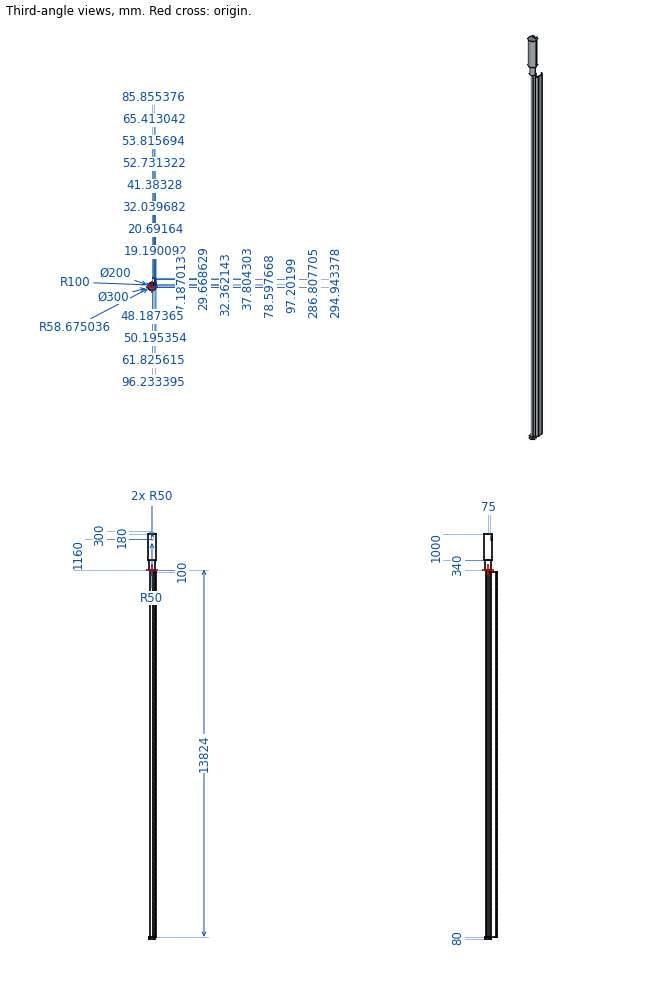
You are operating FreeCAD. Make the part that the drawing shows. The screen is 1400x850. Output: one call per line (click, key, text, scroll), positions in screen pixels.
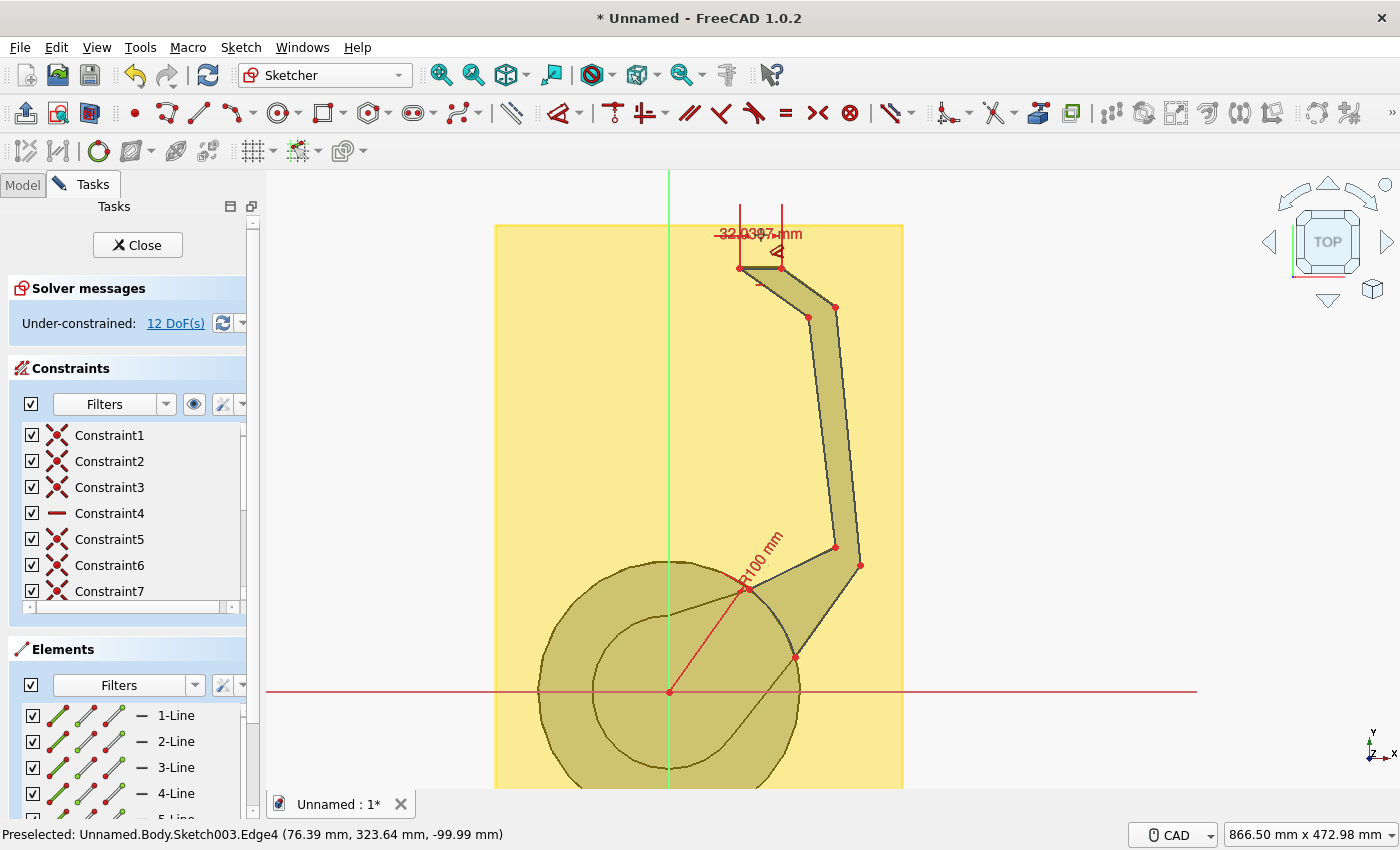
click(861, 566)
click(635, 629)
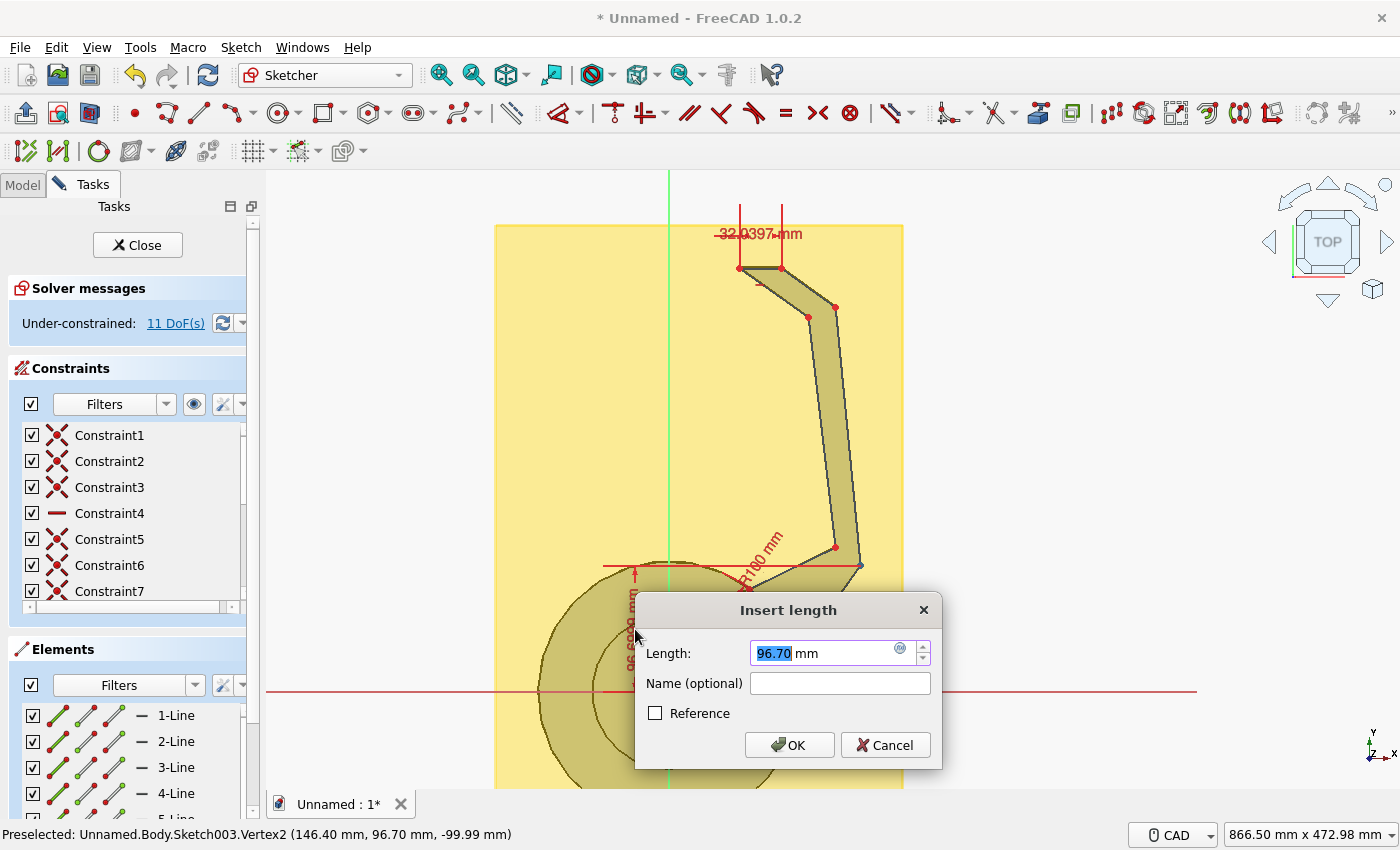
text(97.20199)
key(Return)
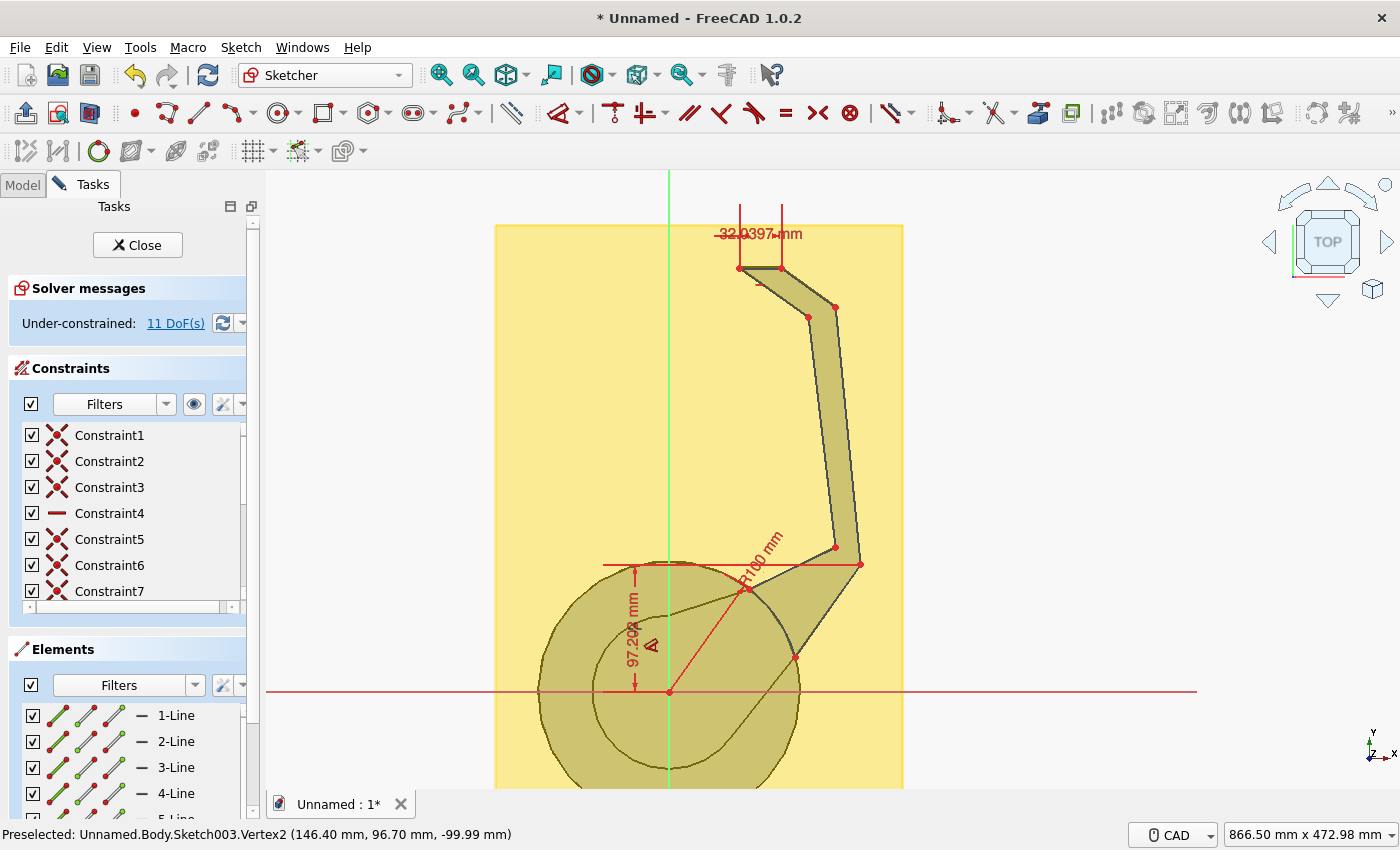
click(819, 296)
click(796, 342)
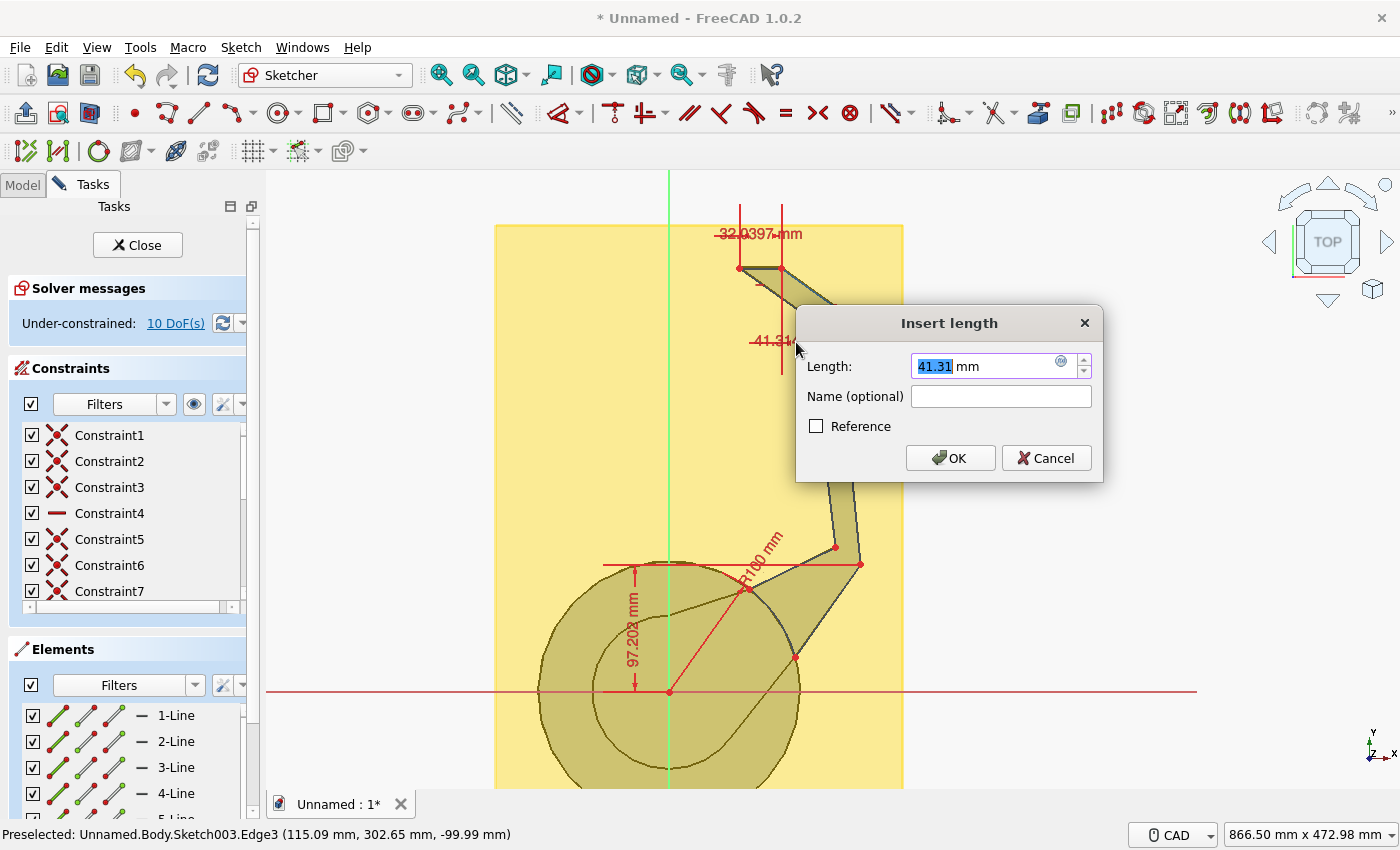
text(41.38328)
key(Return)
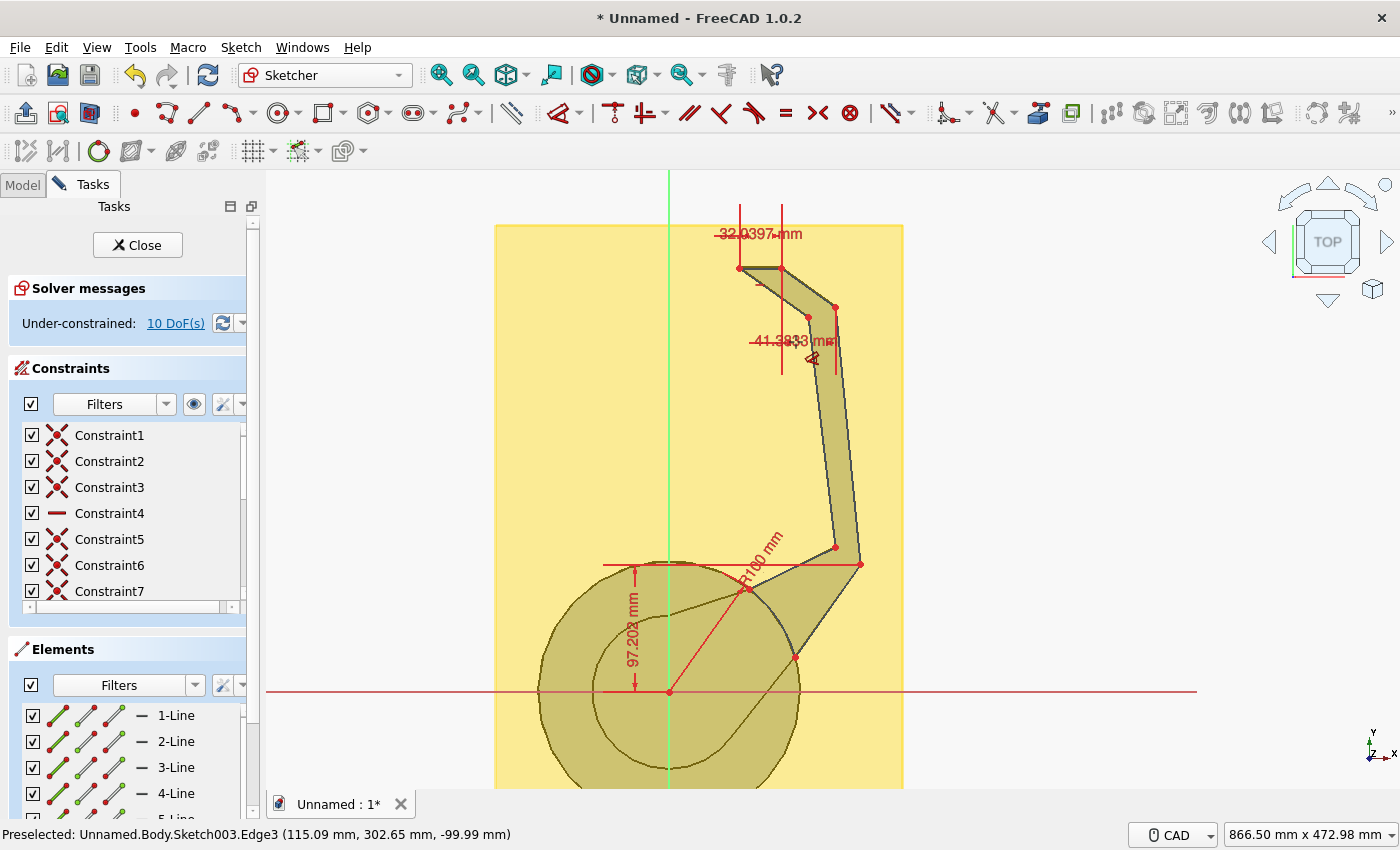
scroll(817, 387, up, 2)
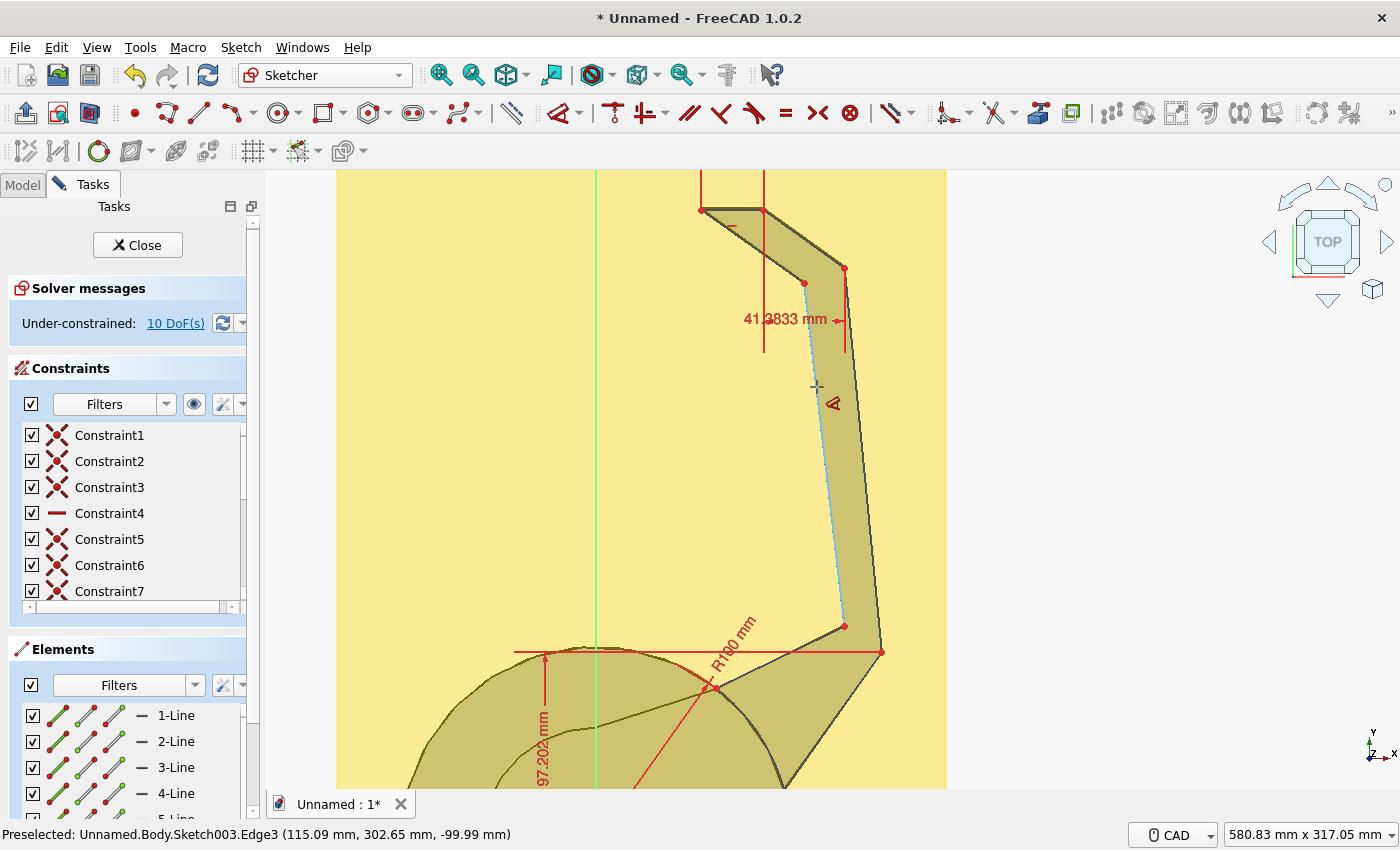
click(816, 386)
click(824, 660)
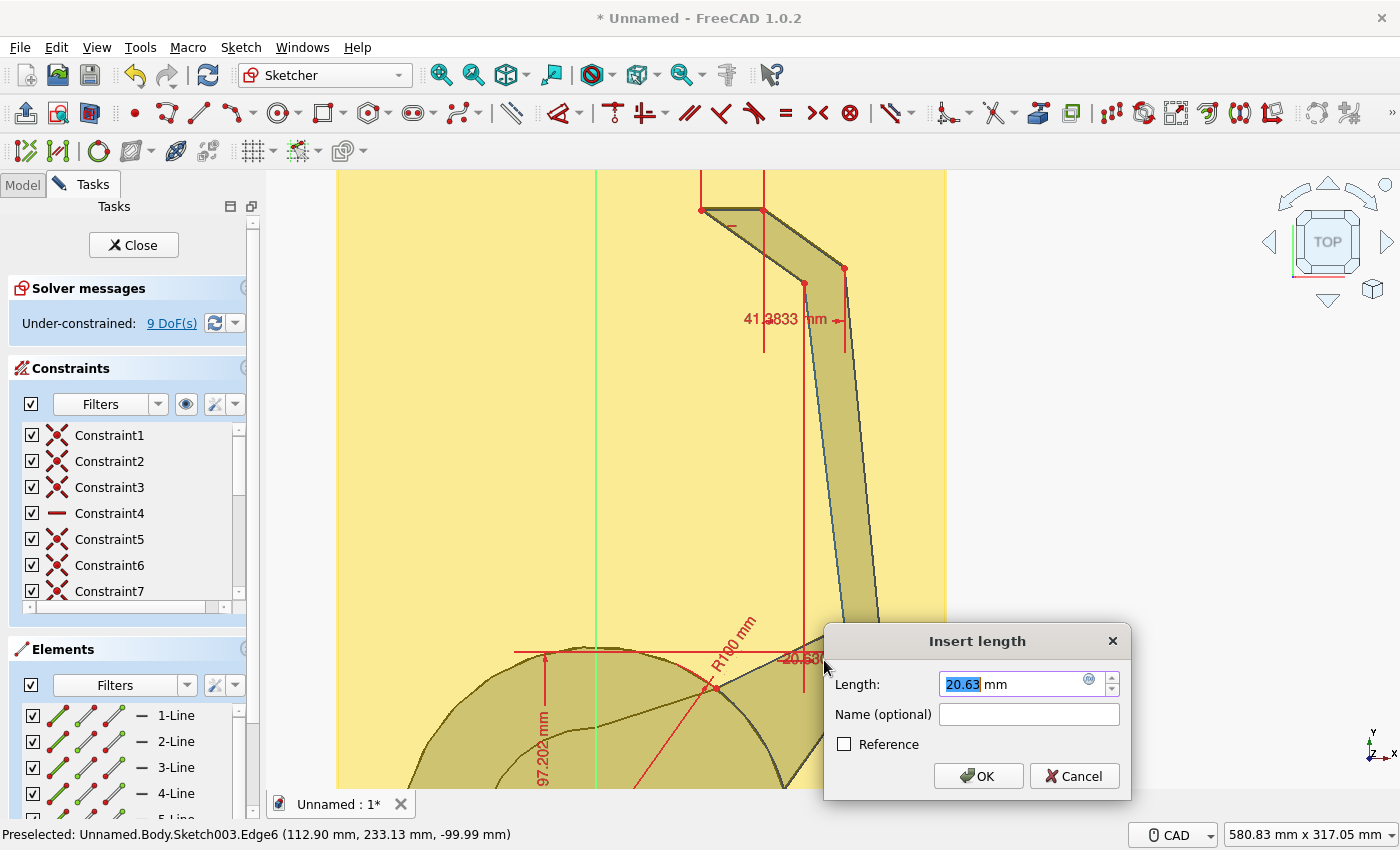
text(20.69164)
key(Return)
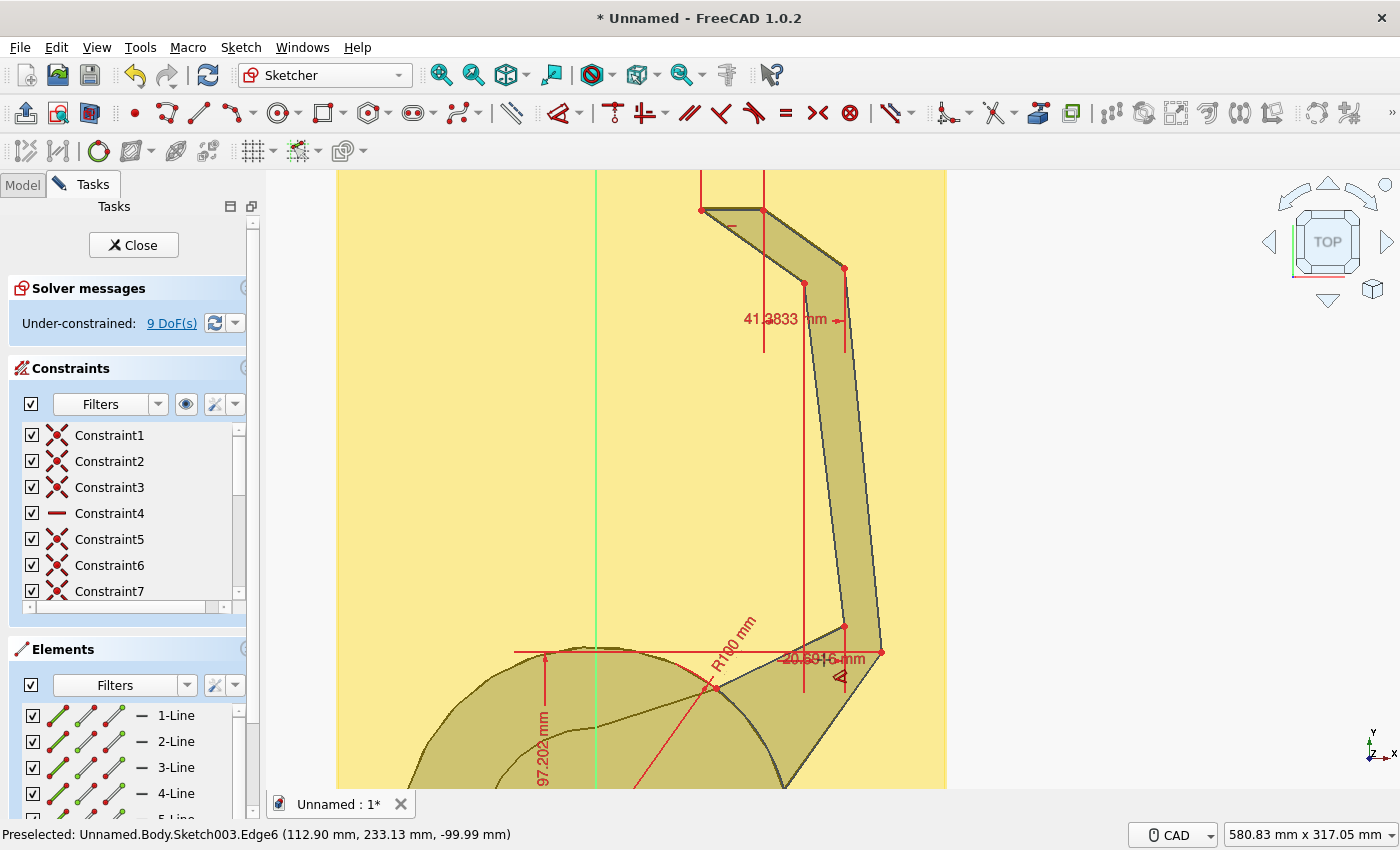
scroll(816, 387, down, 2)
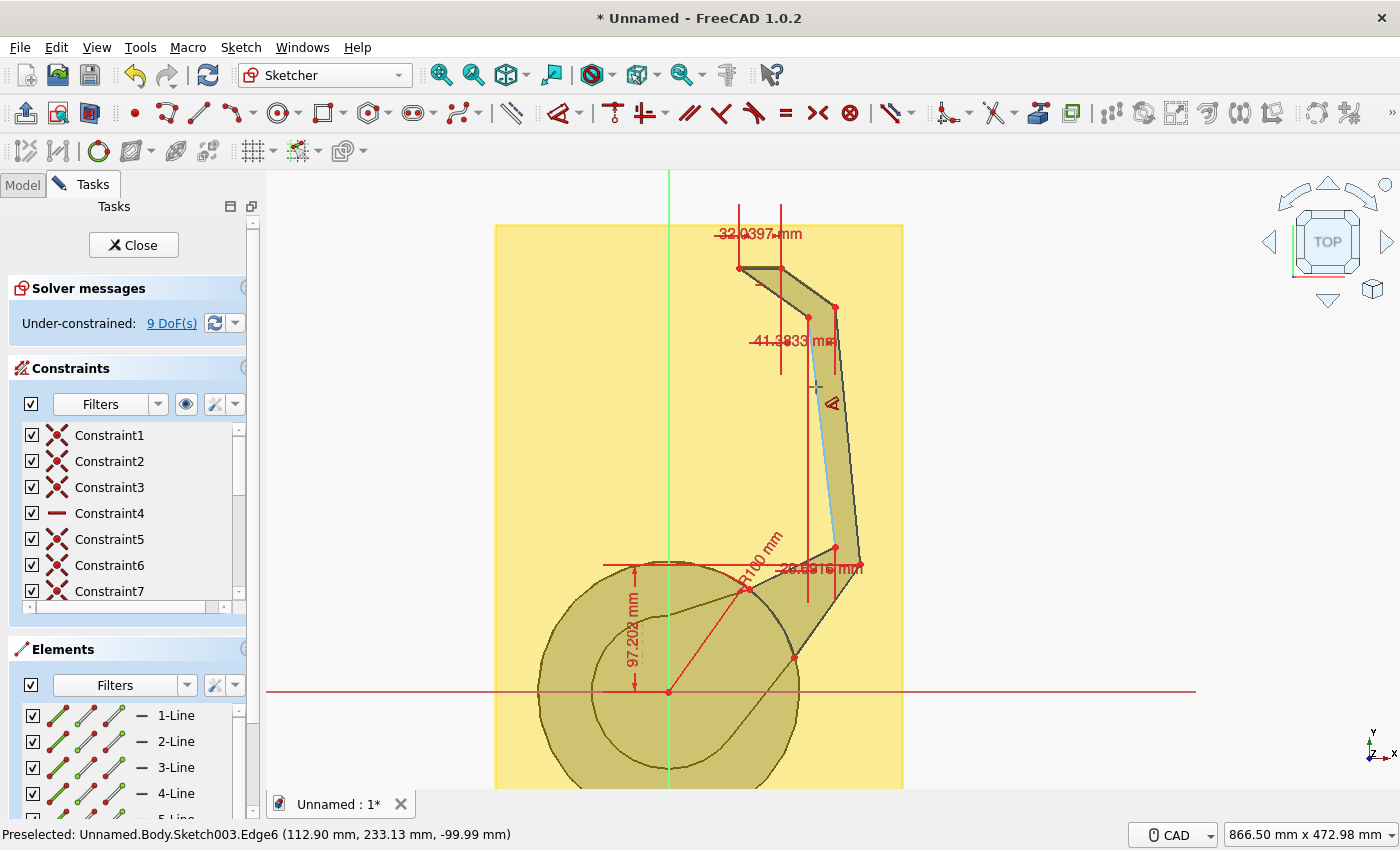
click(795, 658)
click(732, 726)